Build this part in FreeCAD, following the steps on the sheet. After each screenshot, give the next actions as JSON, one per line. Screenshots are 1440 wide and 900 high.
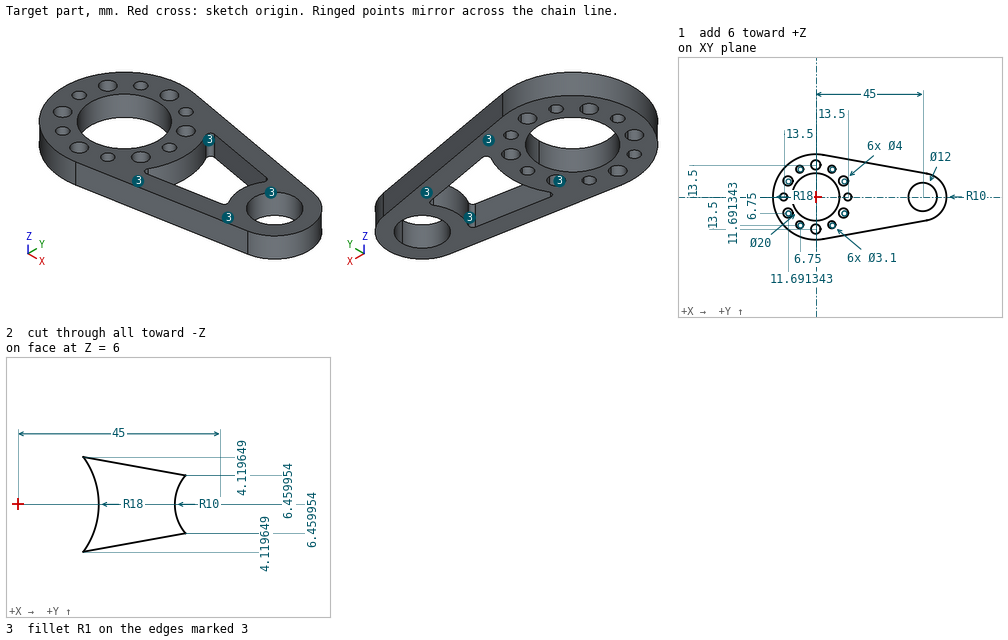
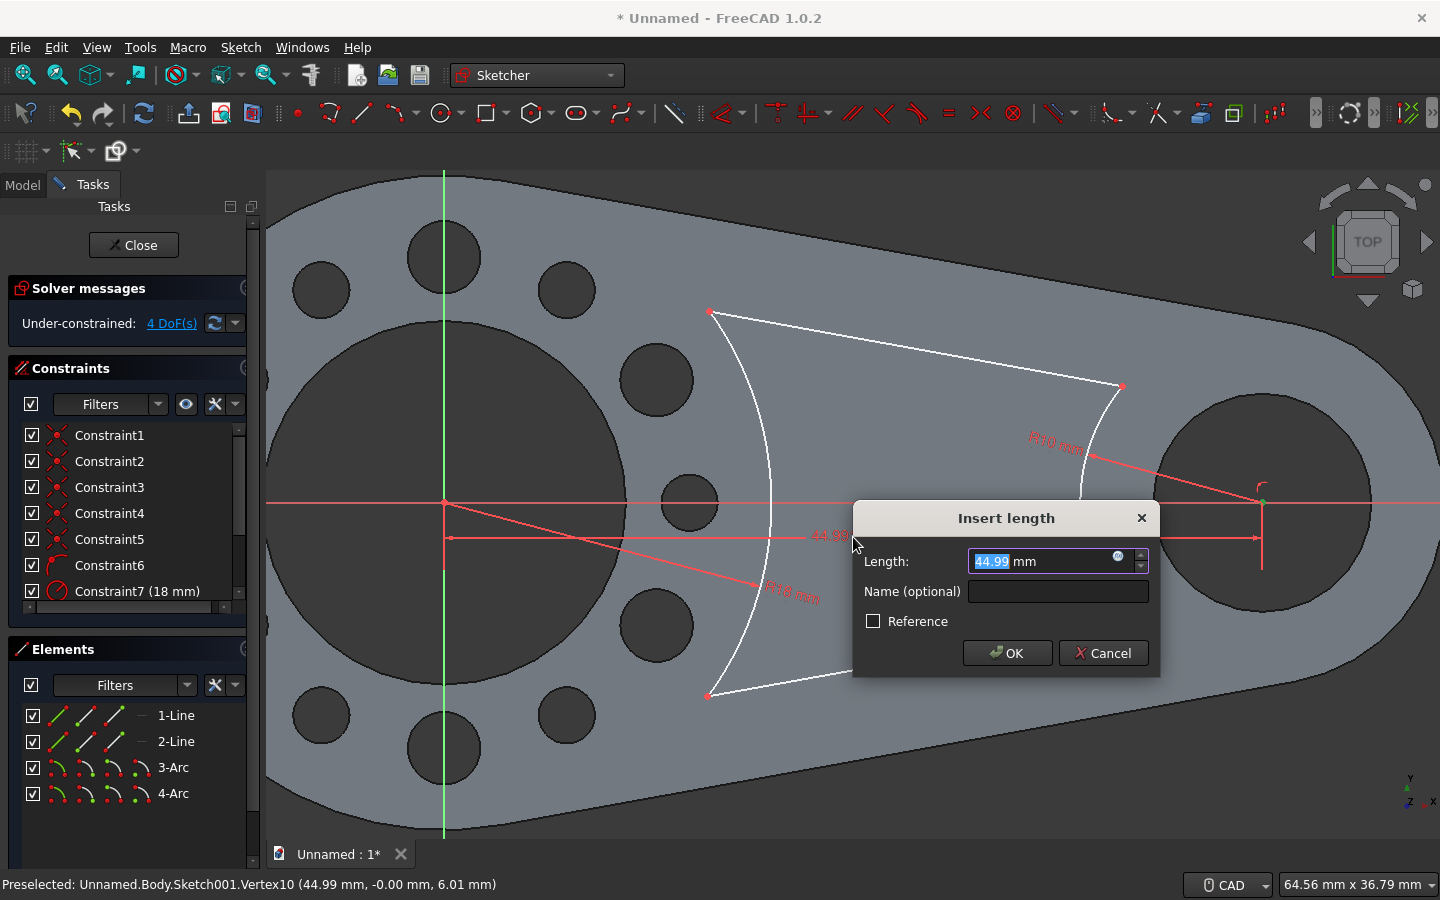
{"action": "type", "text": "45"}
{"action": "key", "text": "Return"}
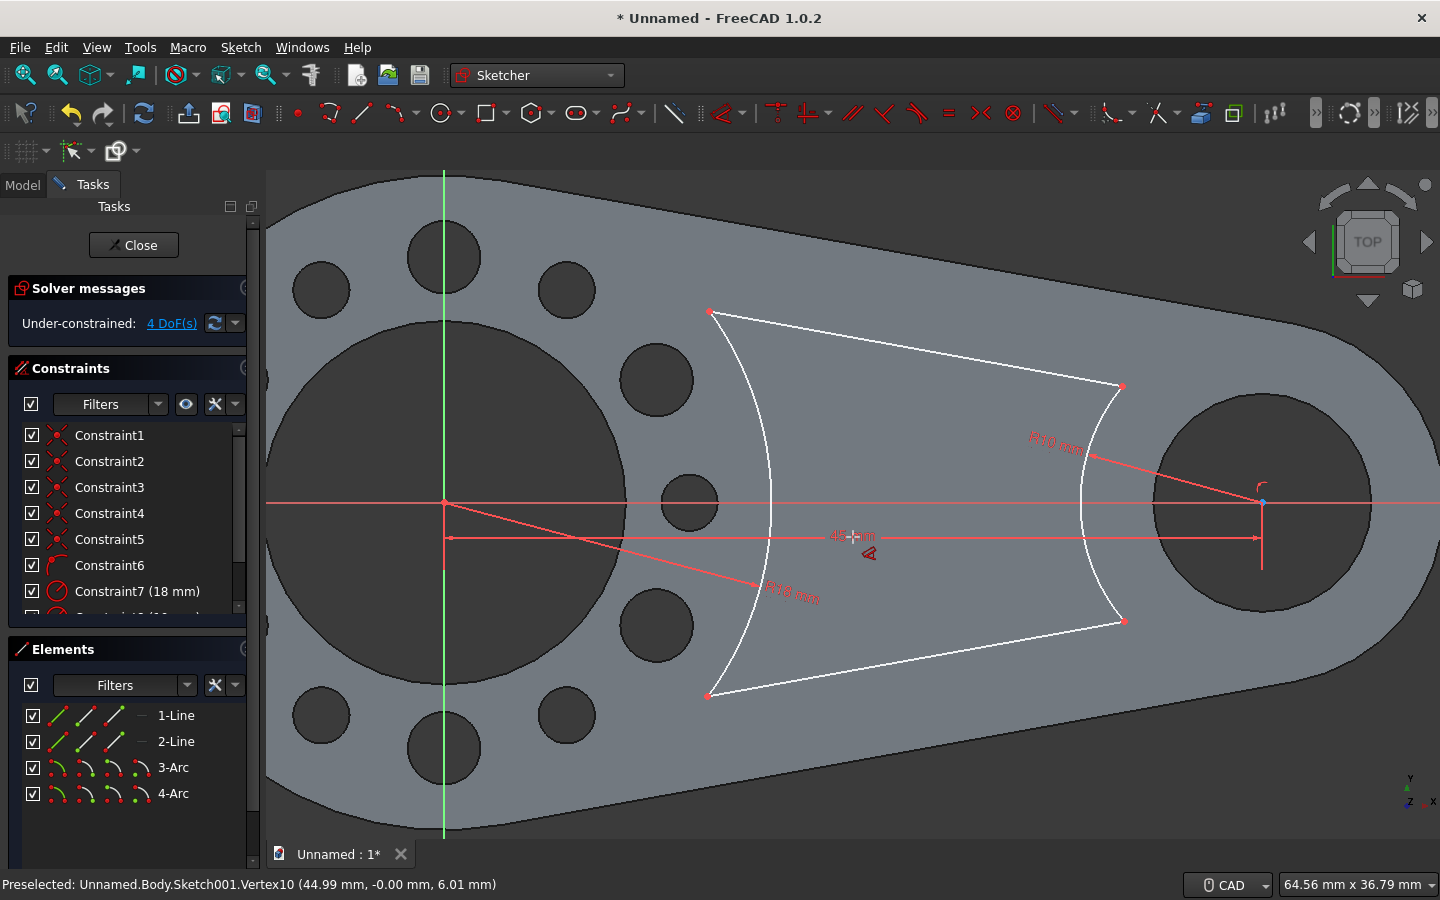
{"action": "left_click", "coordinate": [1123, 386]}
{"action": "left_click", "coordinate": [410, 445]}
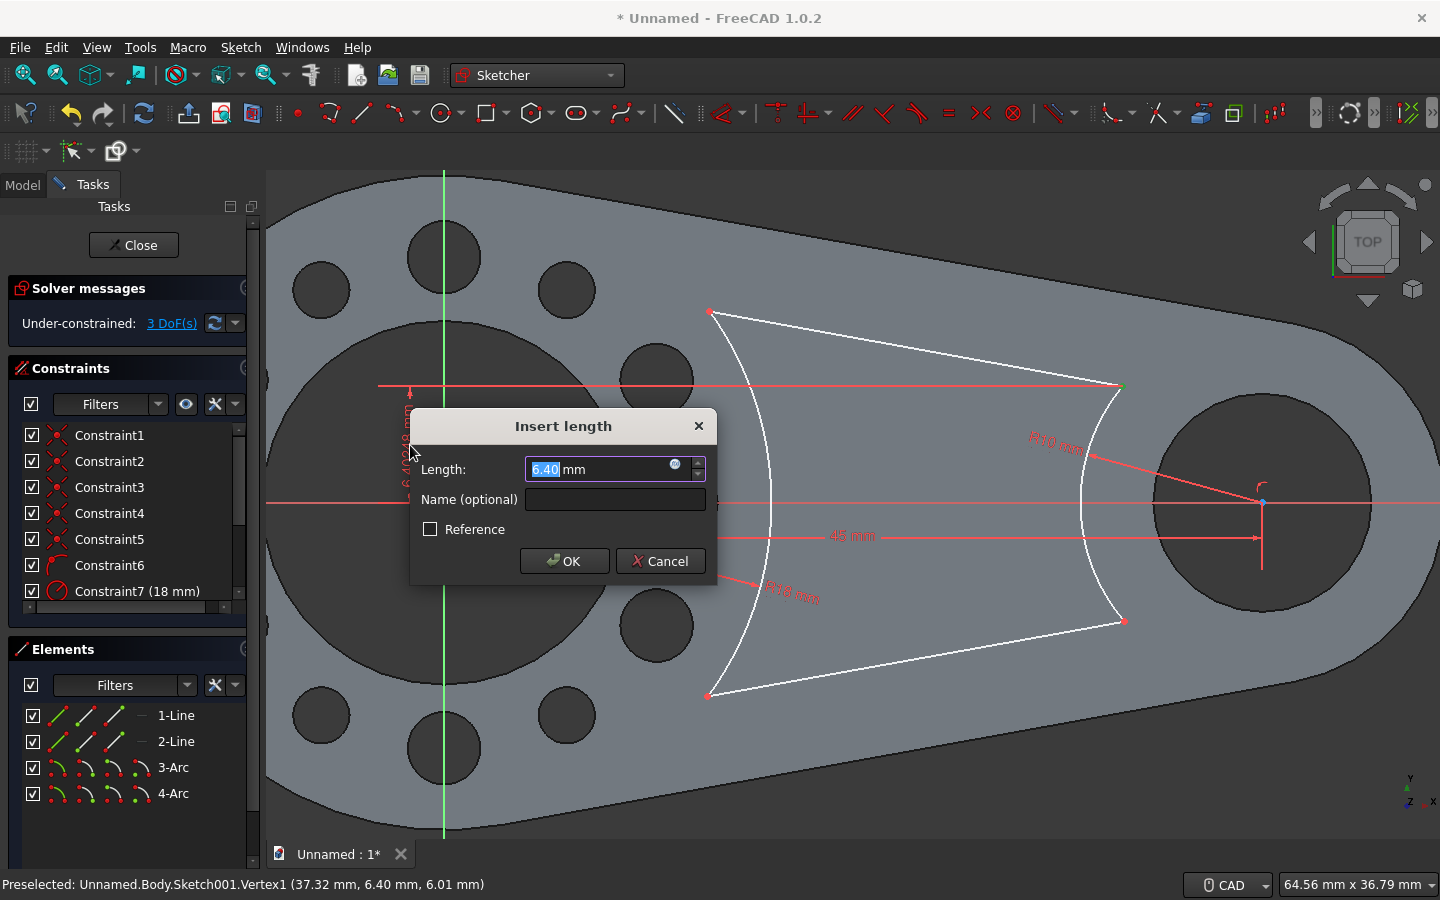
{"action": "type", "text": "6.459954"}
{"action": "key", "text": "Return"}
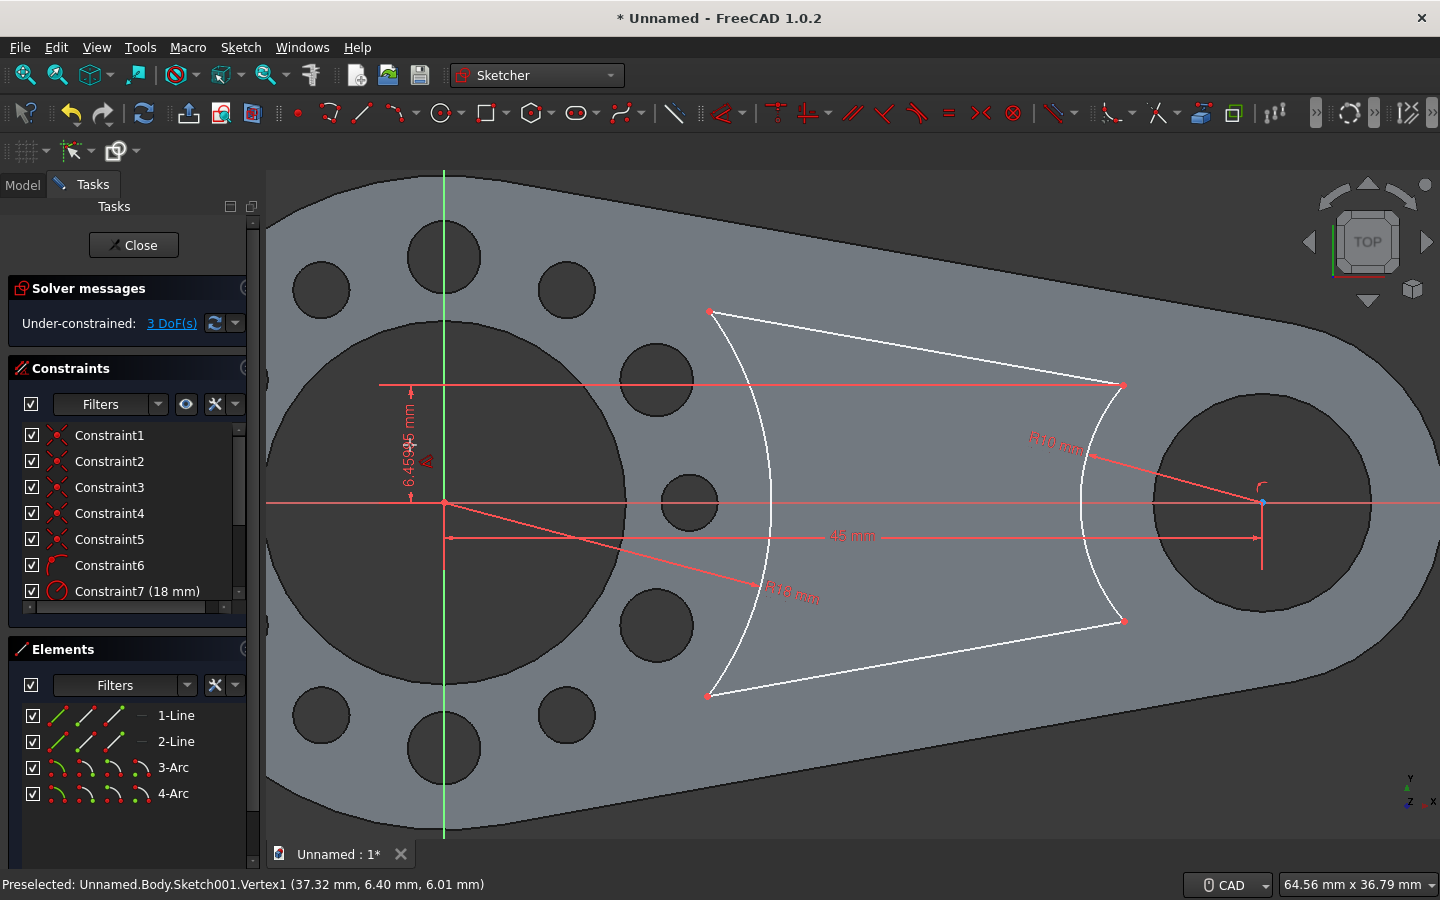
{"action": "left_click", "coordinate": [1125, 622]}
{"action": "left_click", "coordinate": [1159, 562]}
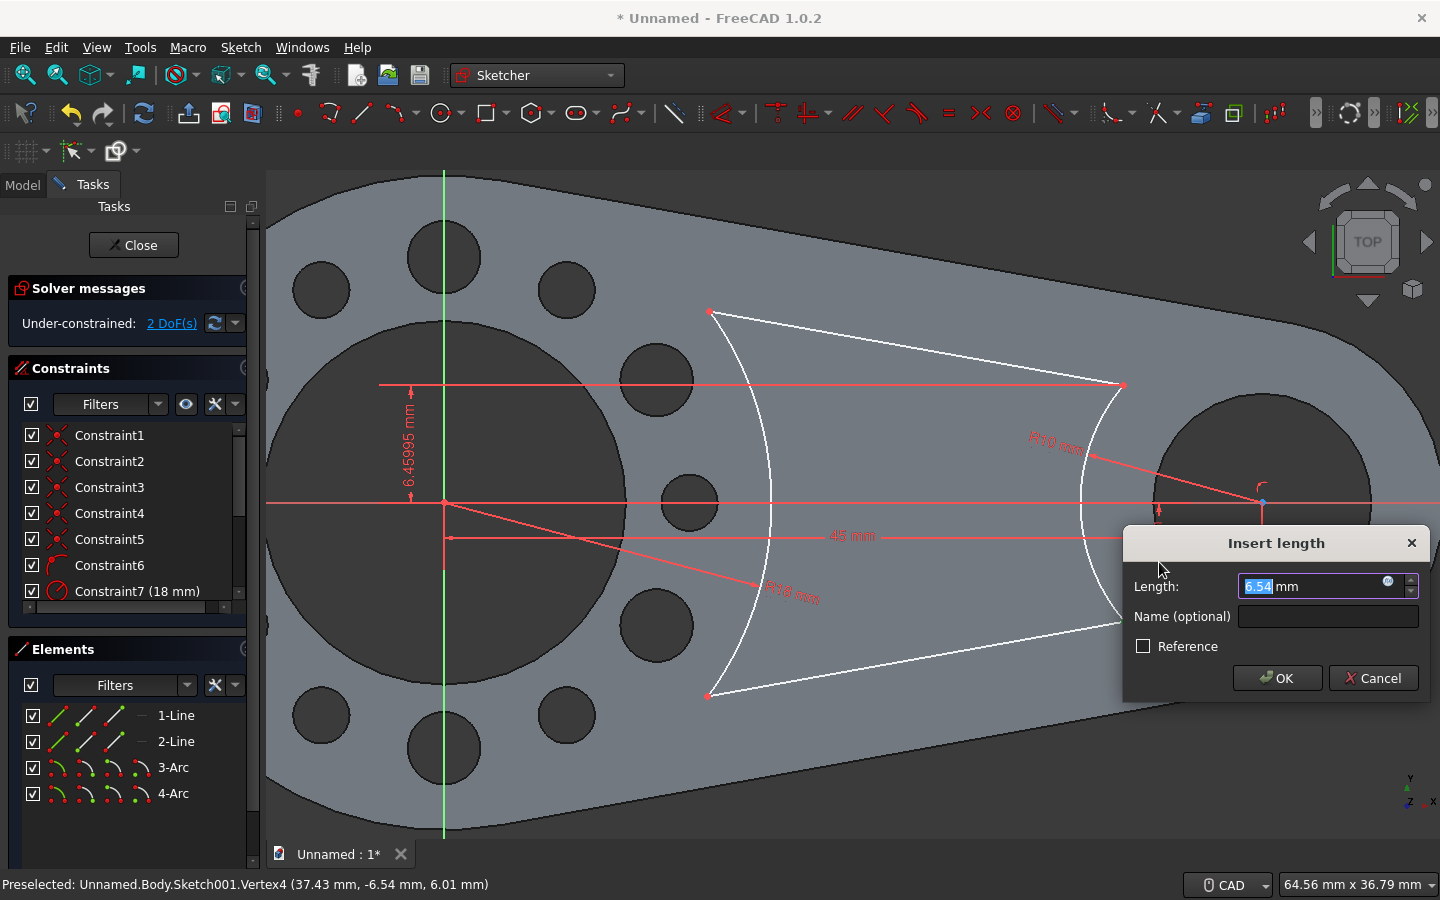
{"action": "type", "text": "6.459954"}
{"action": "key", "text": "Return"}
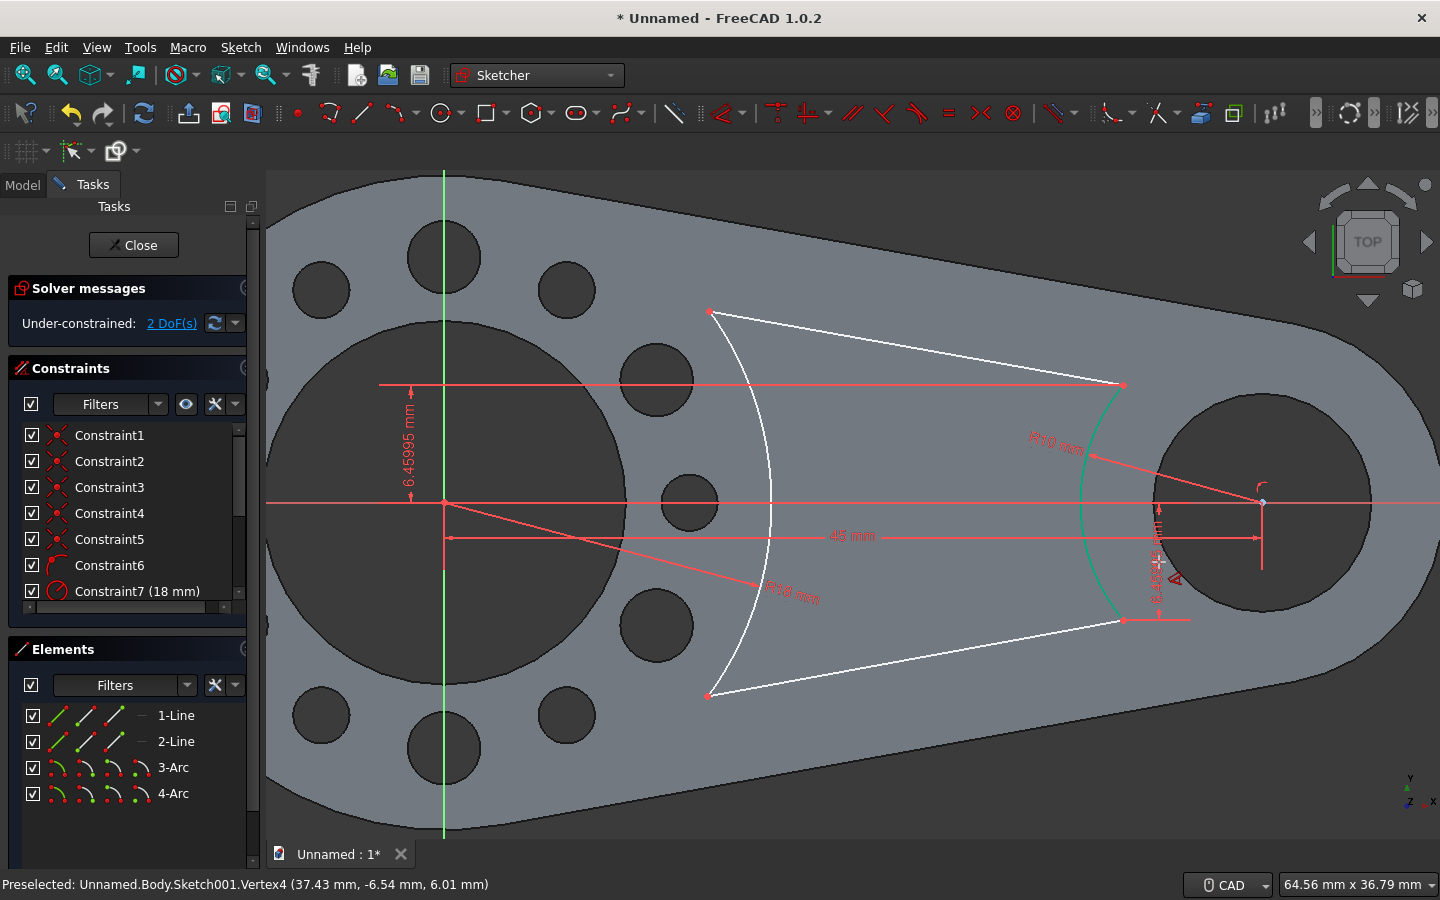
{"action": "left_click", "coordinate": [999, 363]}
{"action": "left_click", "coordinate": [1158, 348]}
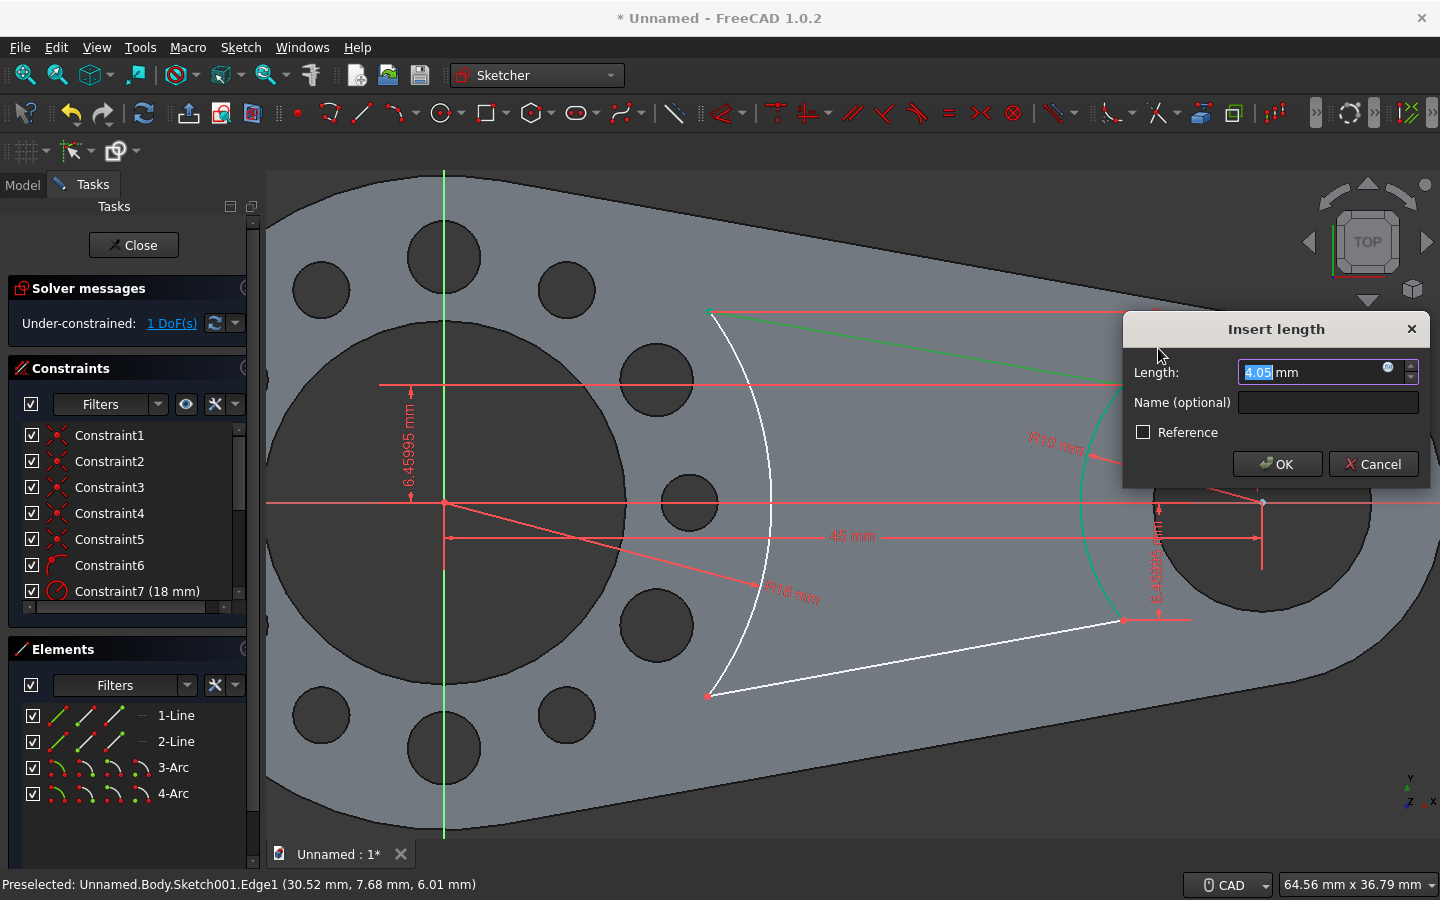
{"action": "type", "text": "4.119649"}
{"action": "key", "text": "Return"}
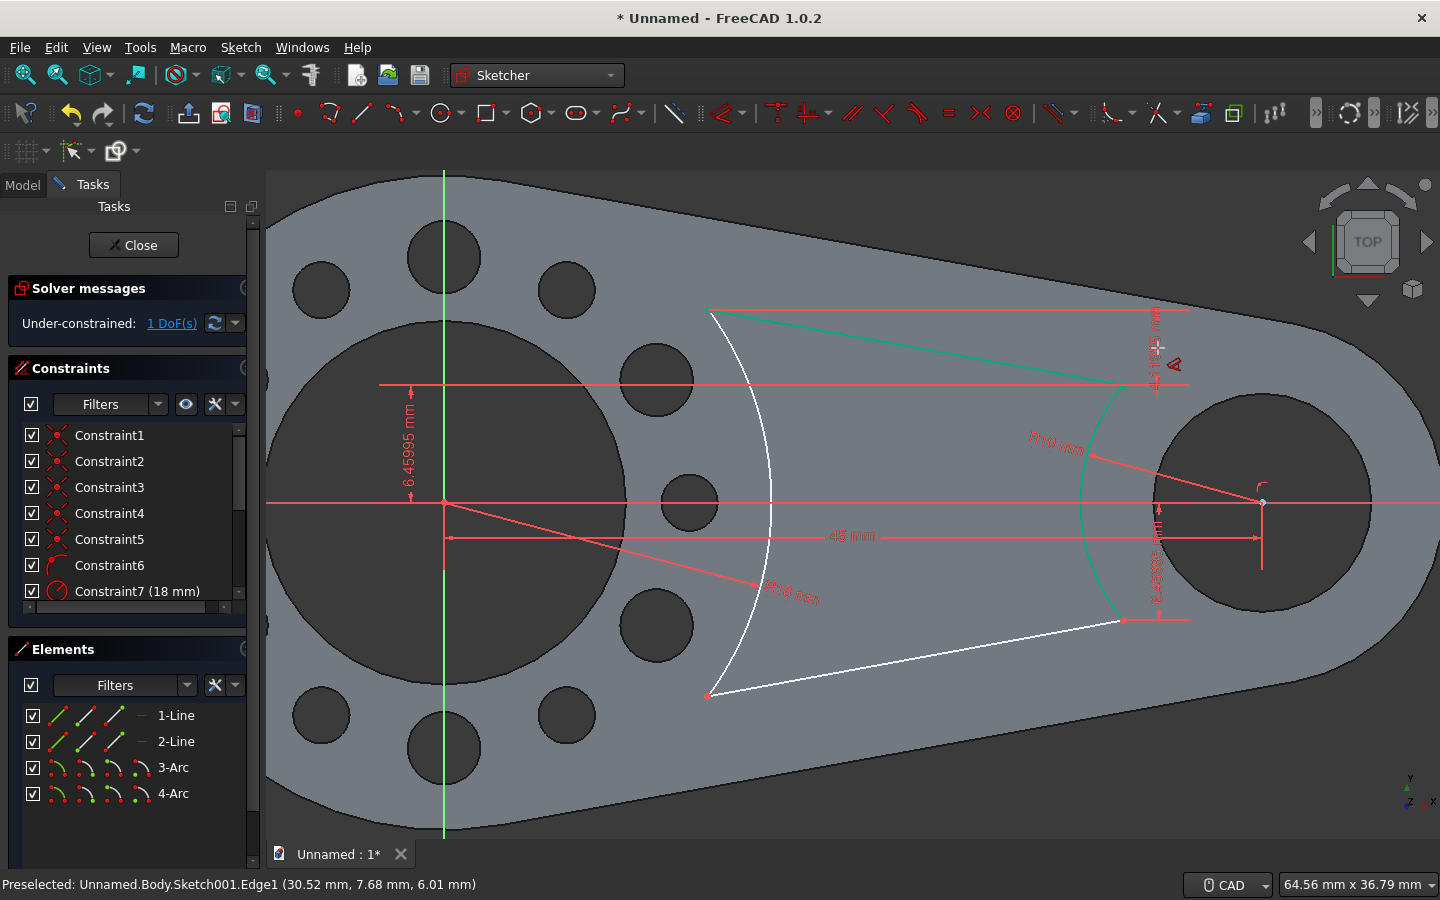
{"action": "left_click", "coordinate": [833, 674]}
{"action": "left_click", "coordinate": [1158, 658]}